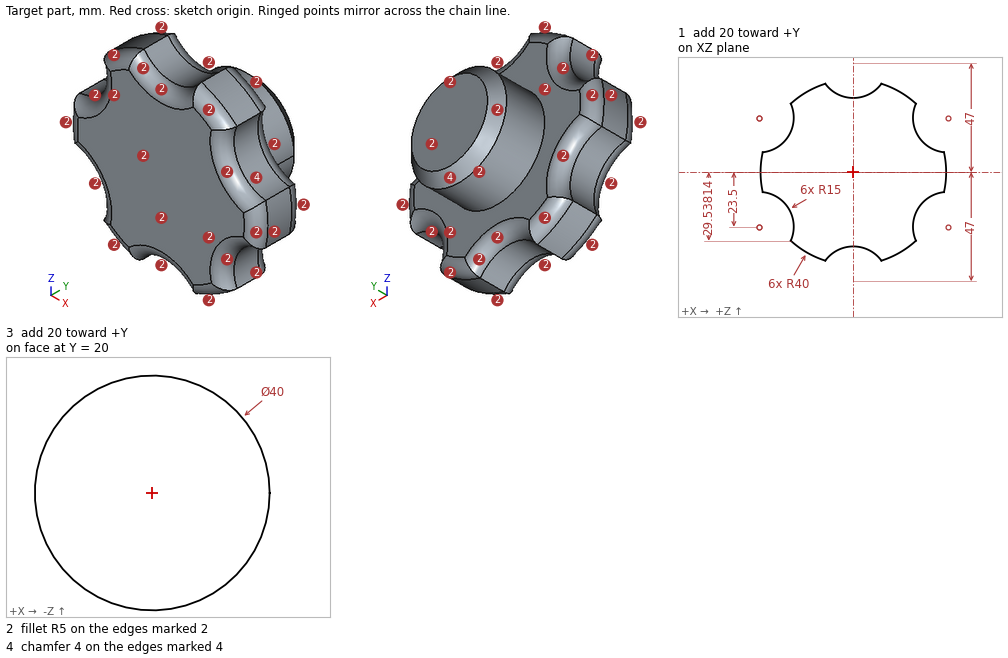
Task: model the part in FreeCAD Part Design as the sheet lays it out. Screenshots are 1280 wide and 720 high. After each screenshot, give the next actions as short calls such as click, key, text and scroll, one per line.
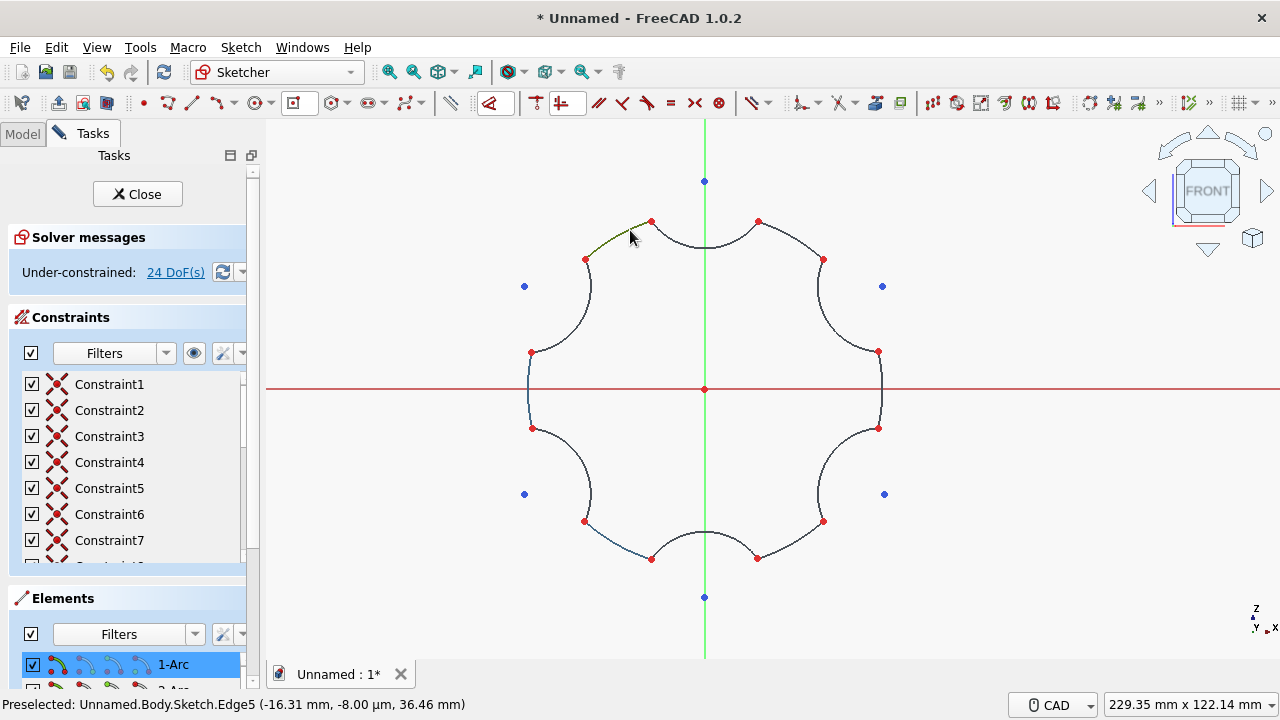
click(806, 246)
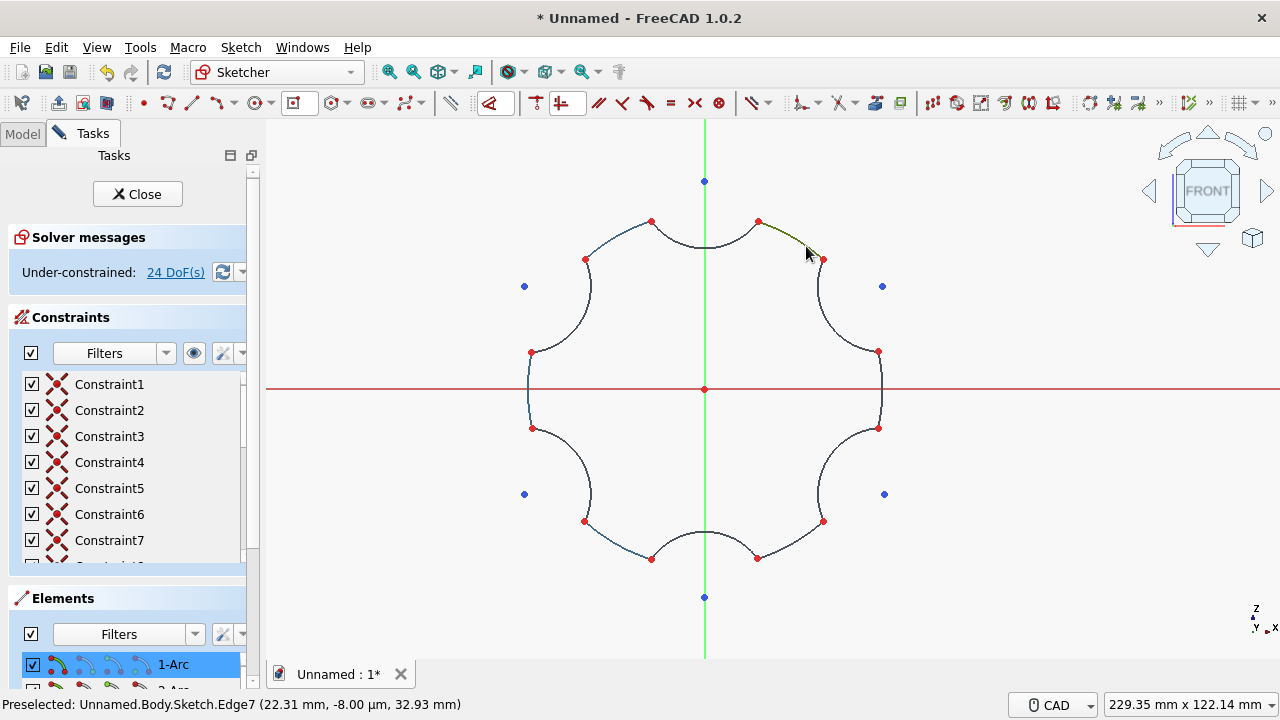
click(882, 405)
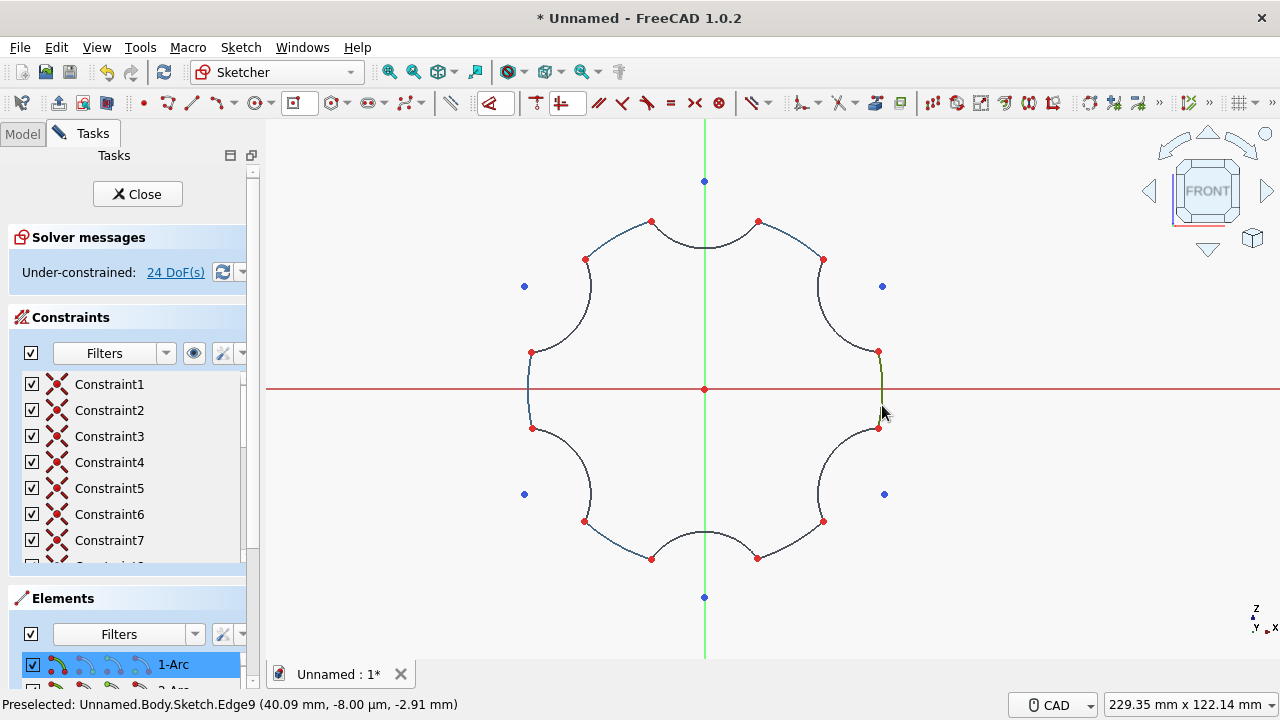
click(779, 551)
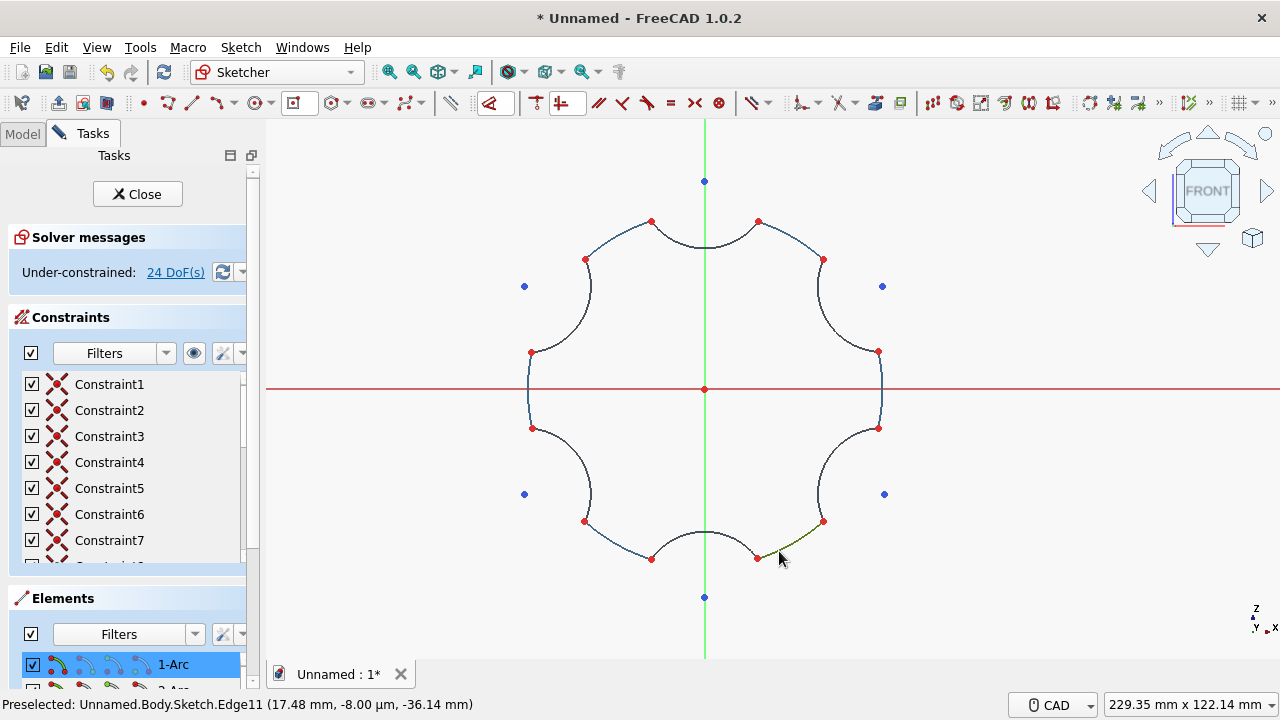
click(672, 104)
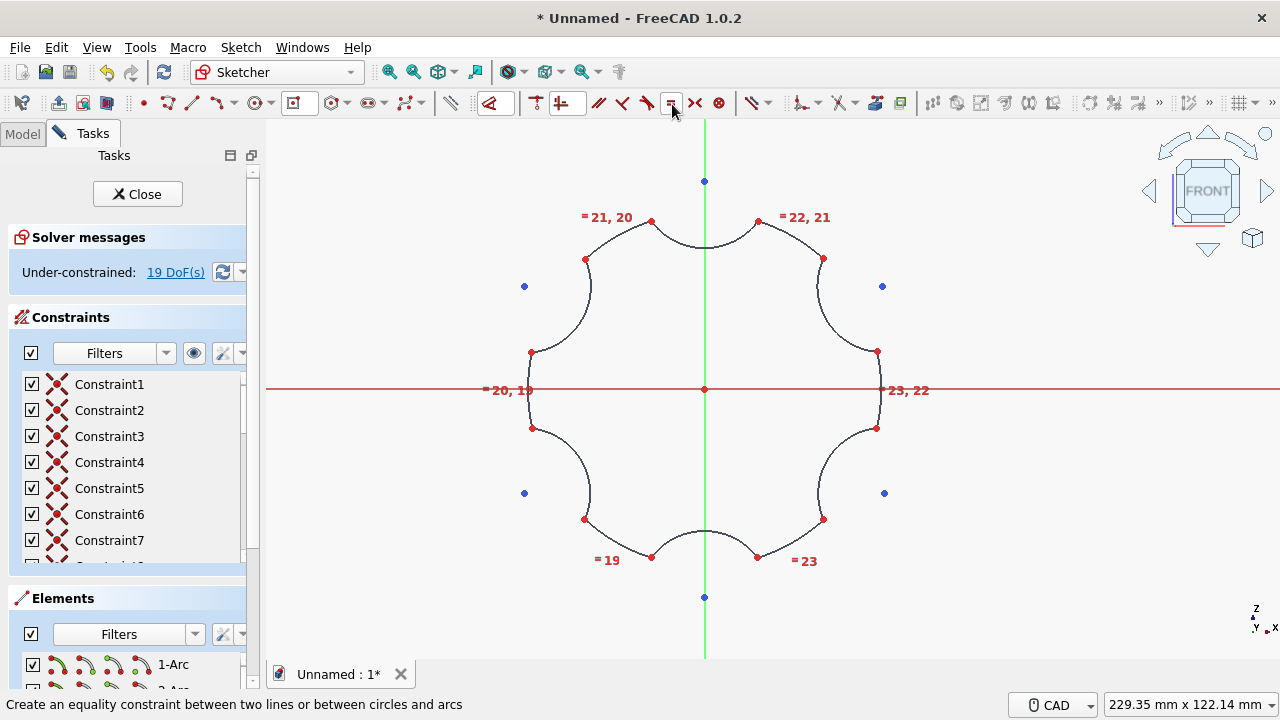
click(589, 484)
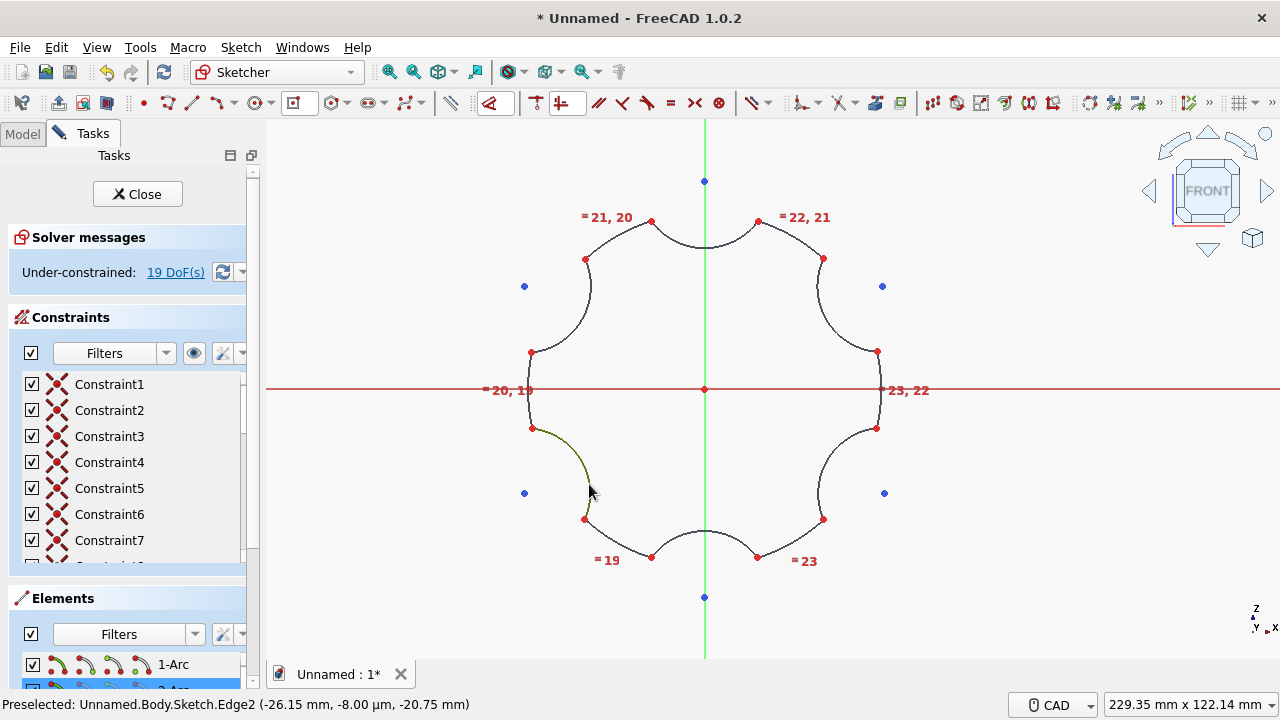
click(566, 338)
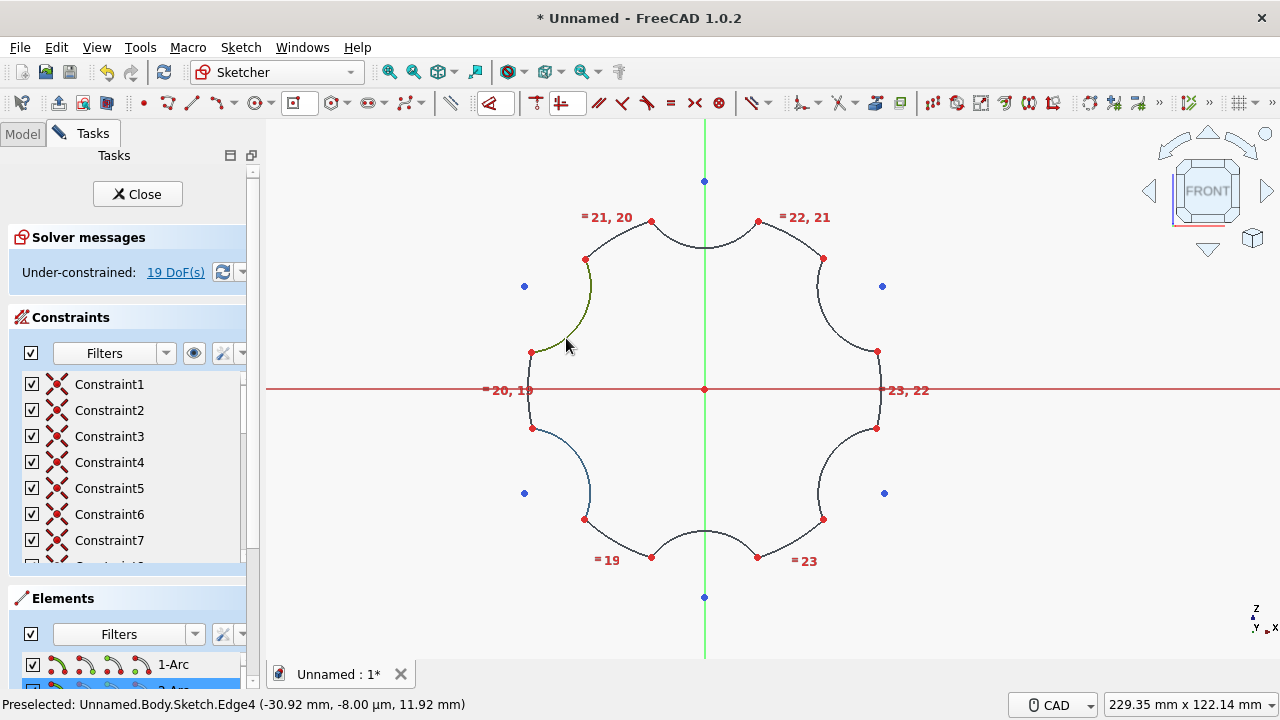
click(680, 244)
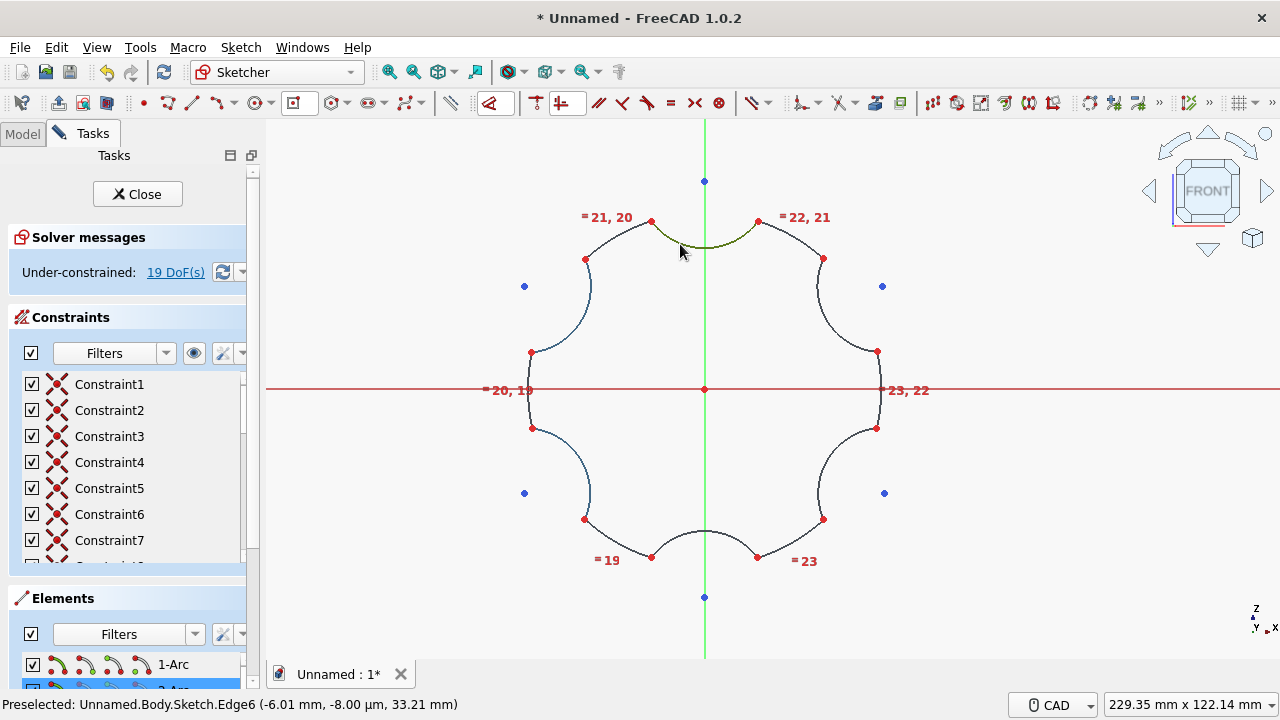
click(818, 296)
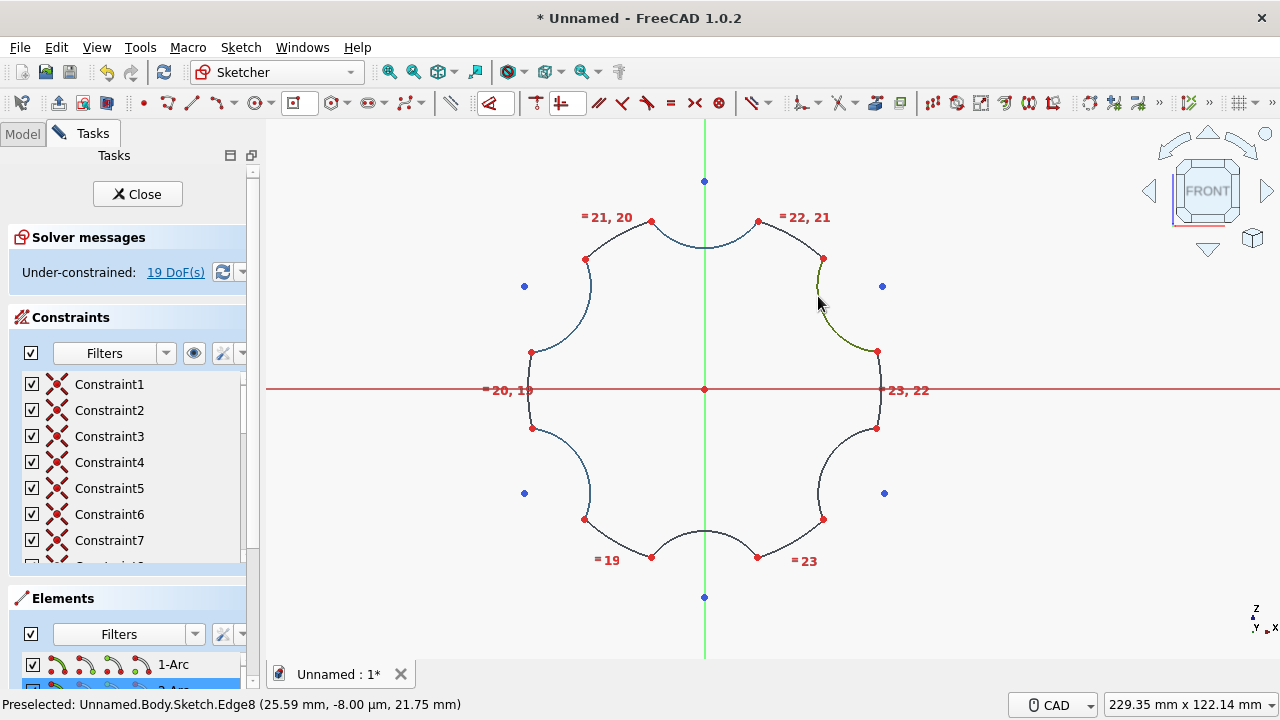
click(843, 442)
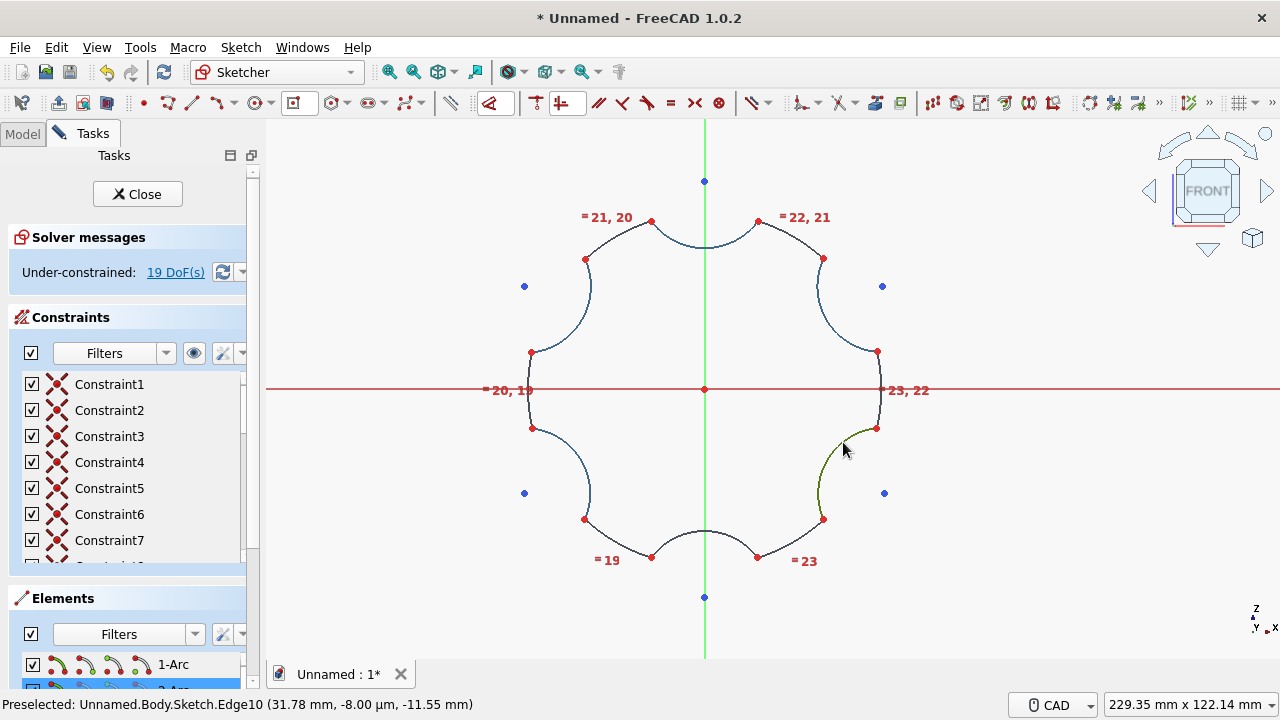
click(729, 536)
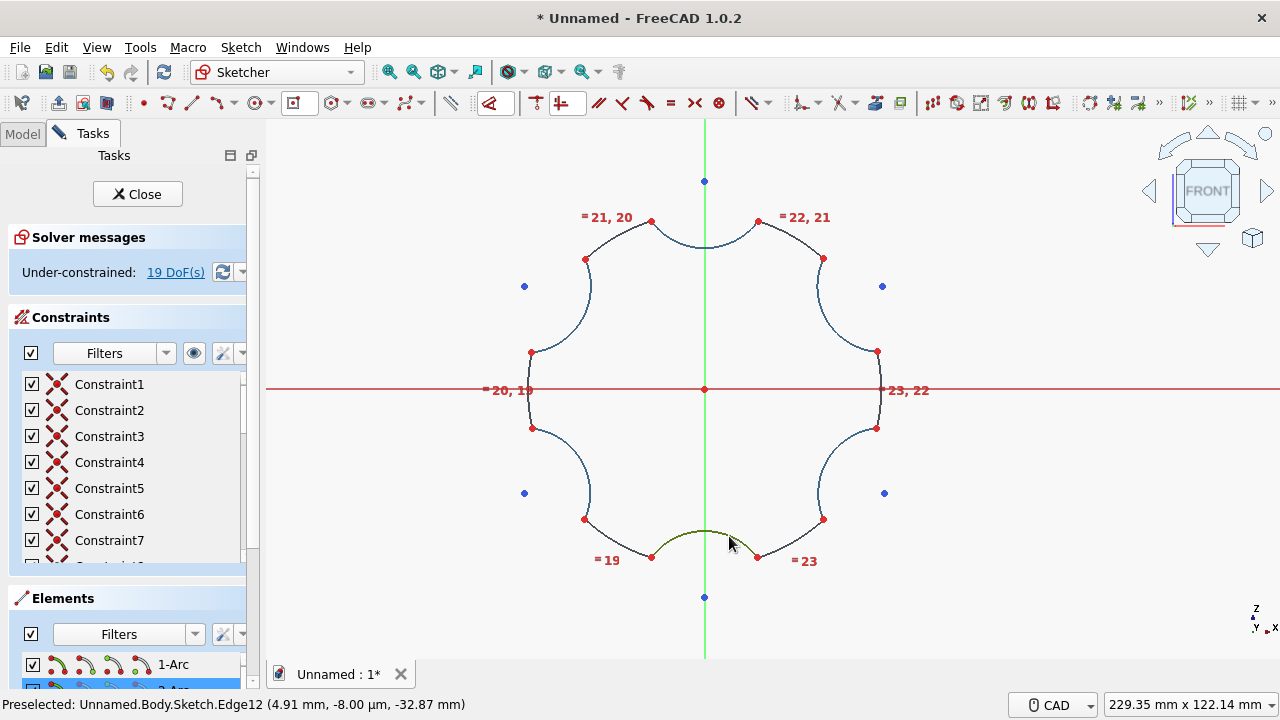
click(672, 104)